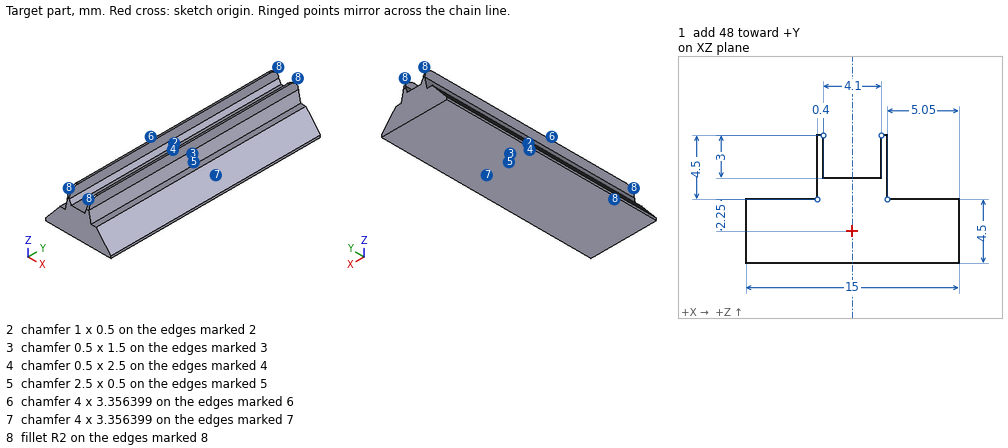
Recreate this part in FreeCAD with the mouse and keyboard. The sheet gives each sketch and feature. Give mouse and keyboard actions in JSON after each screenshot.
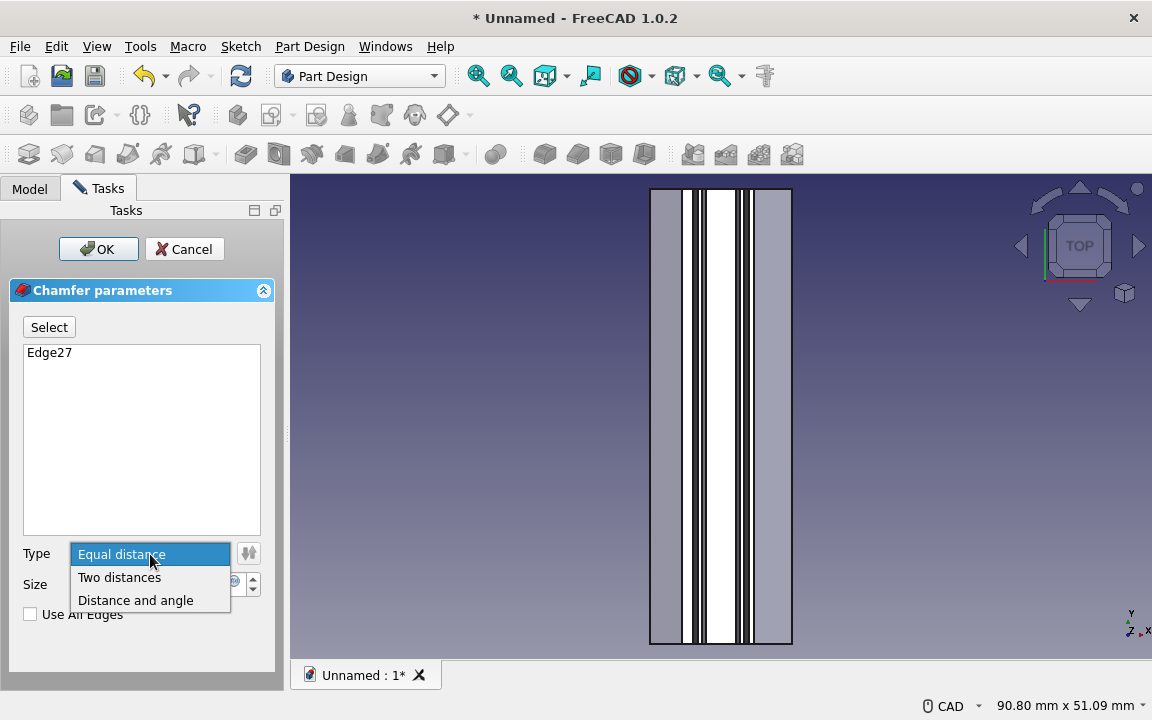
{"action": "left_click", "coordinate": [148, 578]}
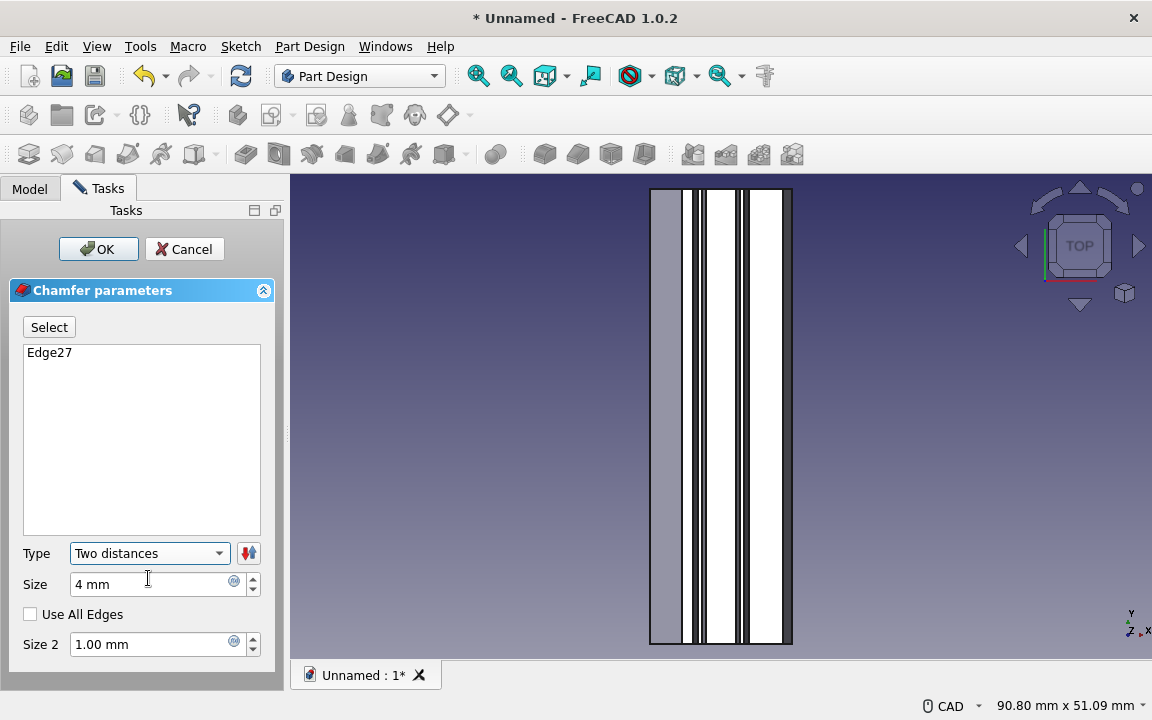
{"action": "triple_click", "coordinate": [158, 644]}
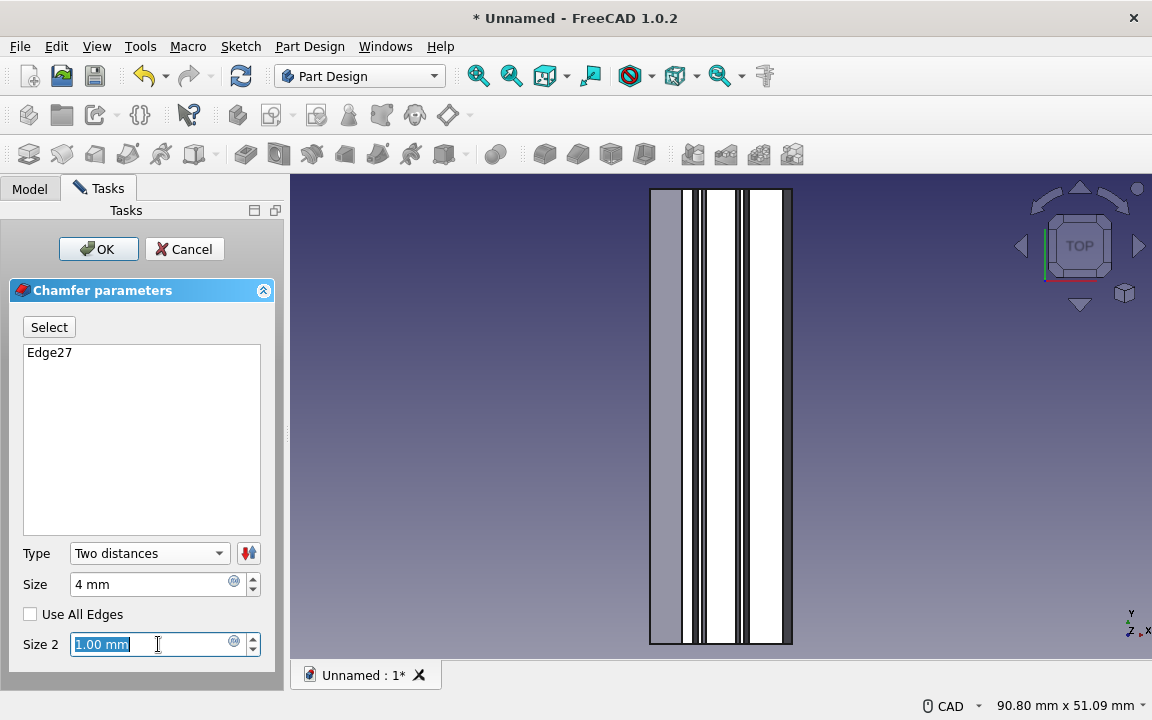
{"action": "type", "text": "3.356399"}
{"action": "key", "text": "Tab"}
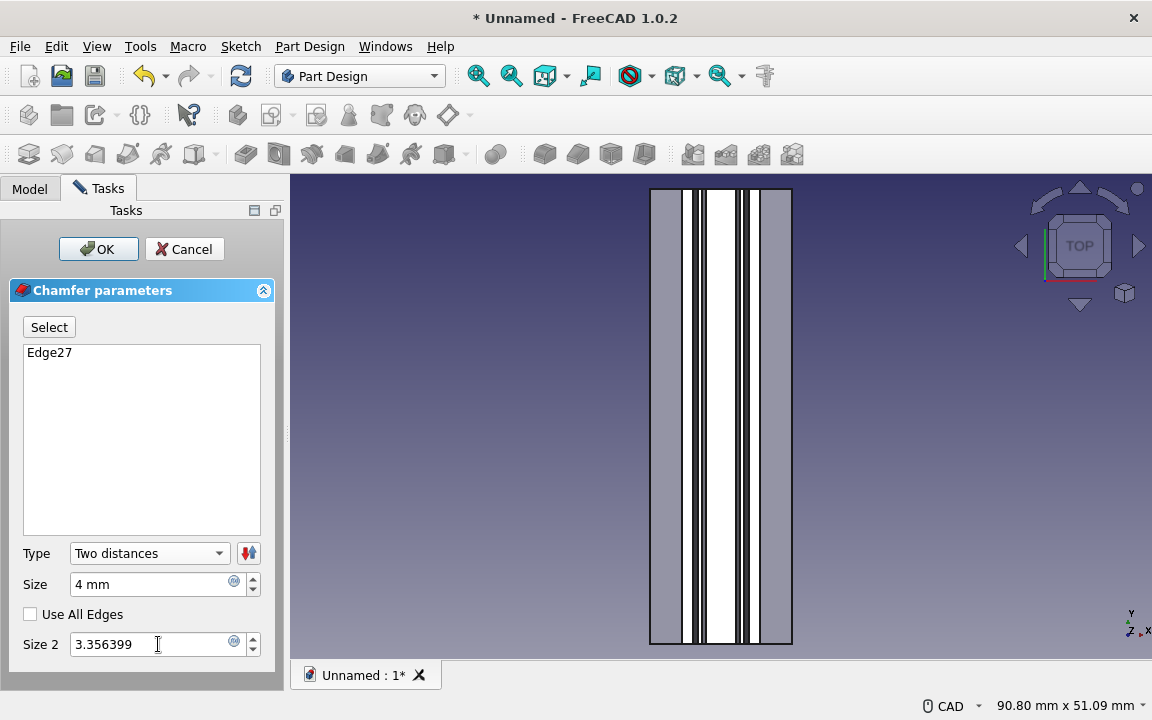
{"action": "left_click", "coordinate": [99, 249]}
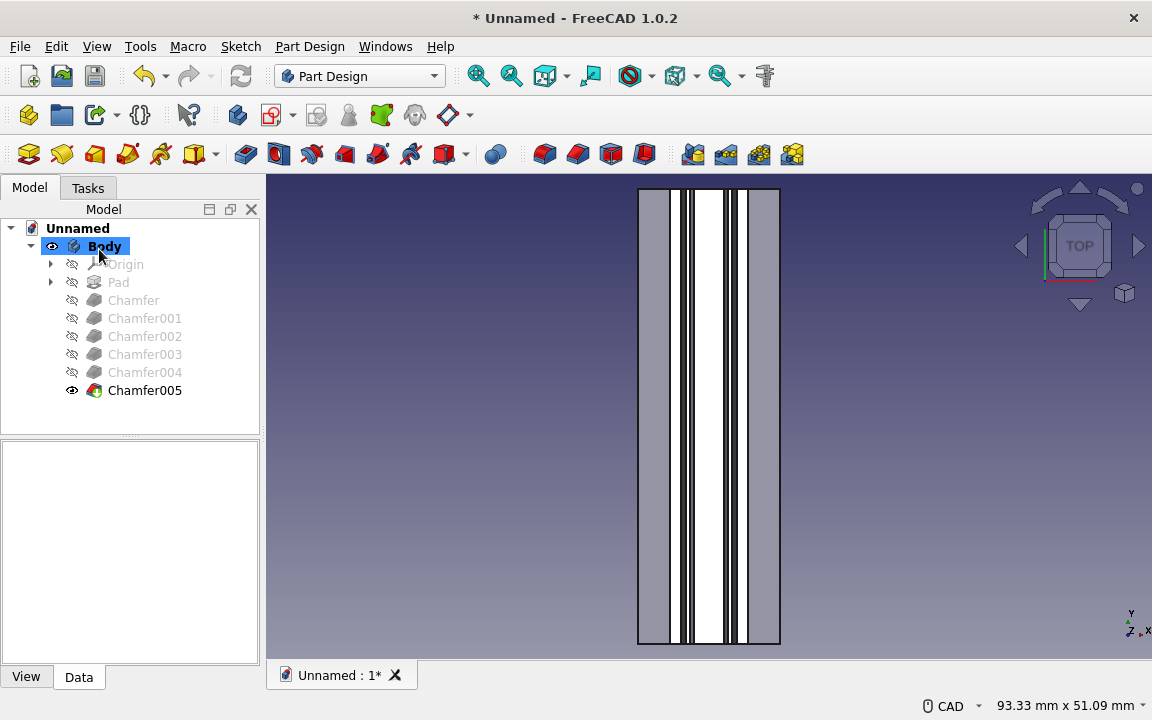
{"action": "key", "text": "0"}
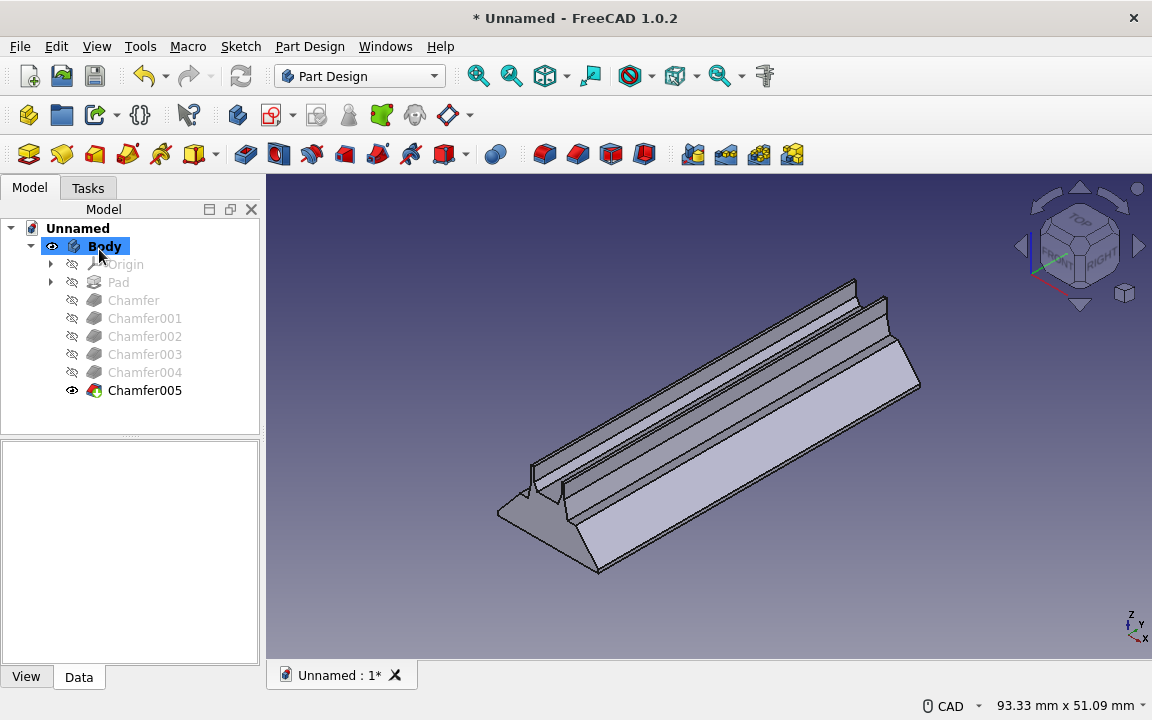
{"action": "scroll", "coordinate": [533, 465], "scroll_direction": "up", "scroll_amount": 12}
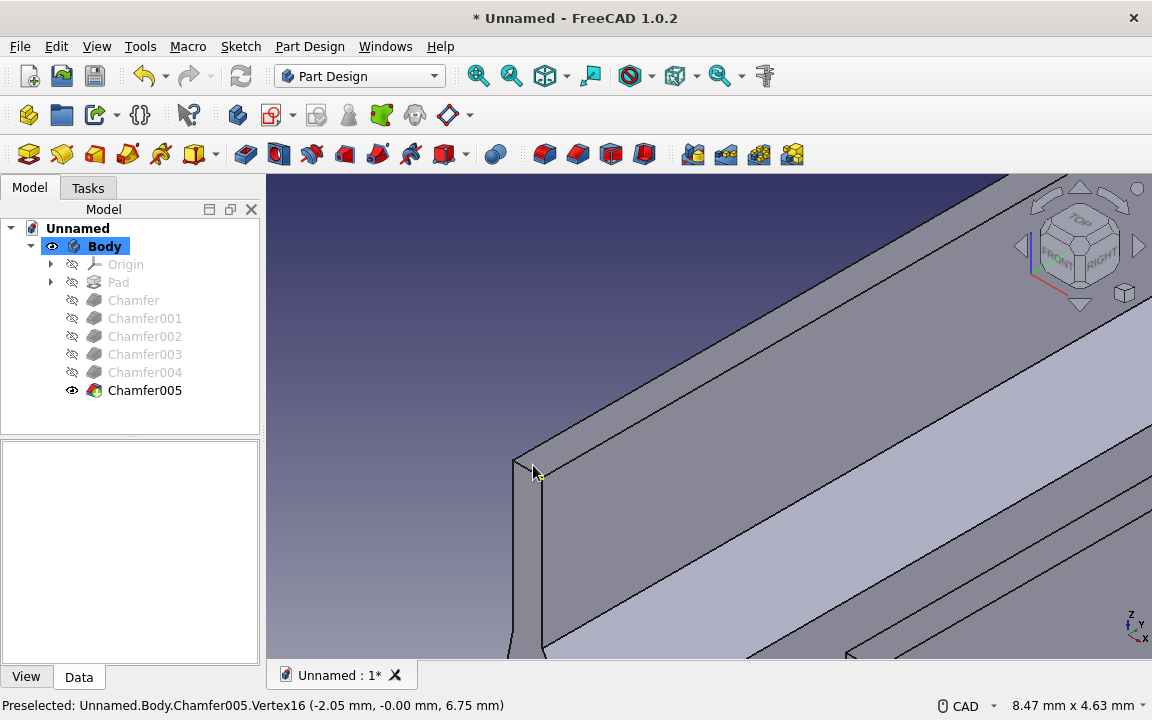
{"action": "left_click", "coordinate": [528, 468]}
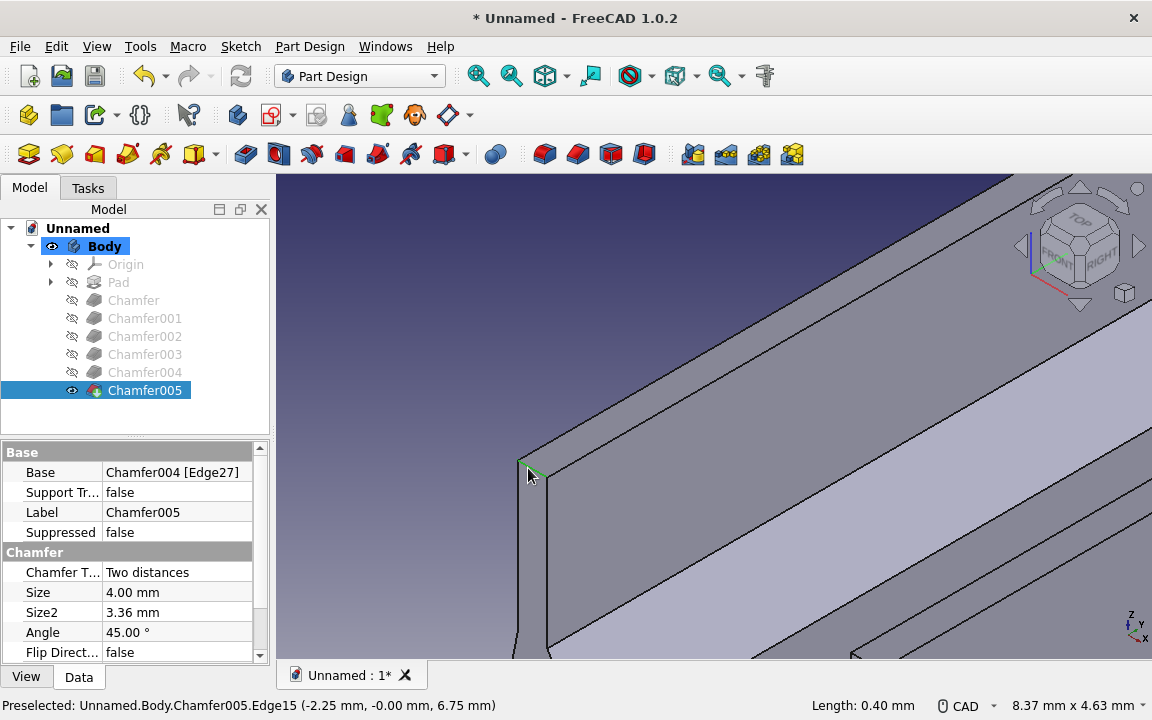
{"action": "key", "text": "v f"}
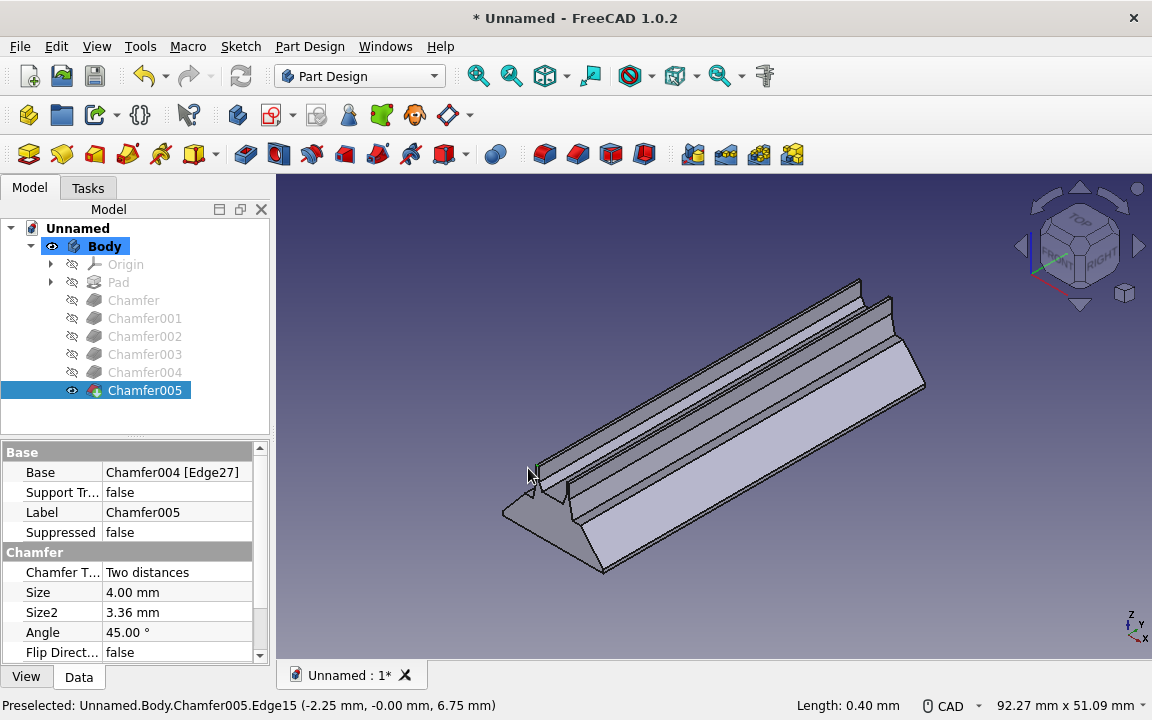
{"action": "key", "text": "2"}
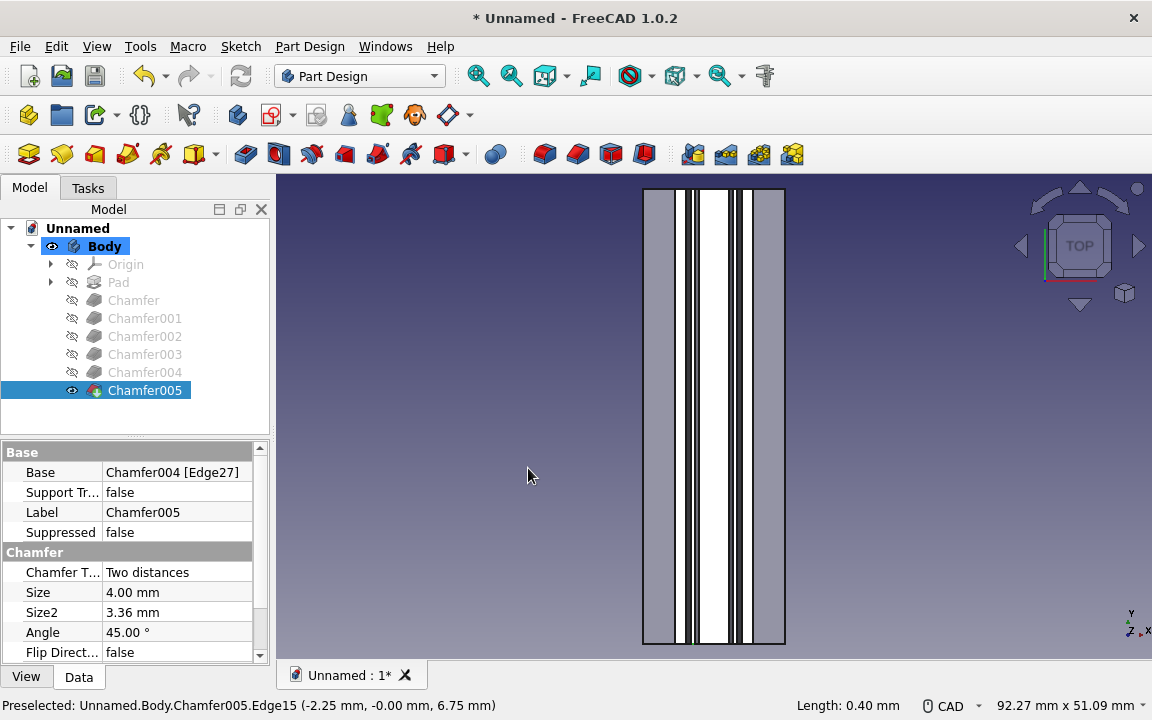
{"action": "key", "text": "1"}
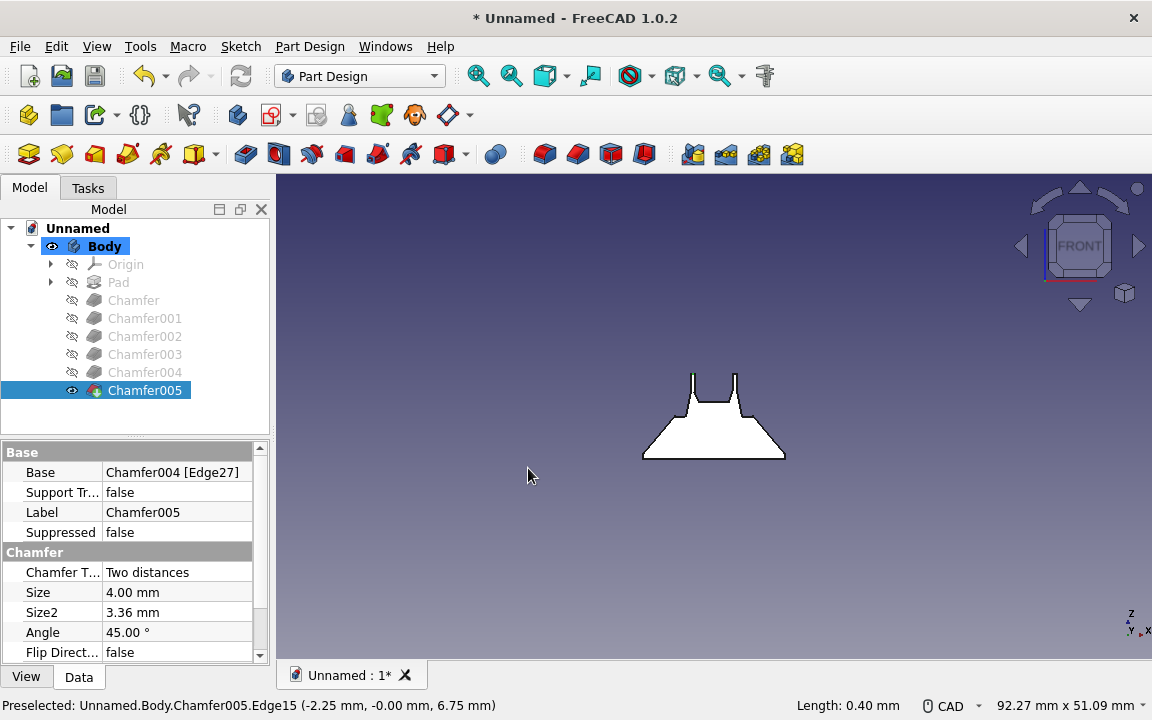
{"action": "left_click", "coordinate": [479, 76]}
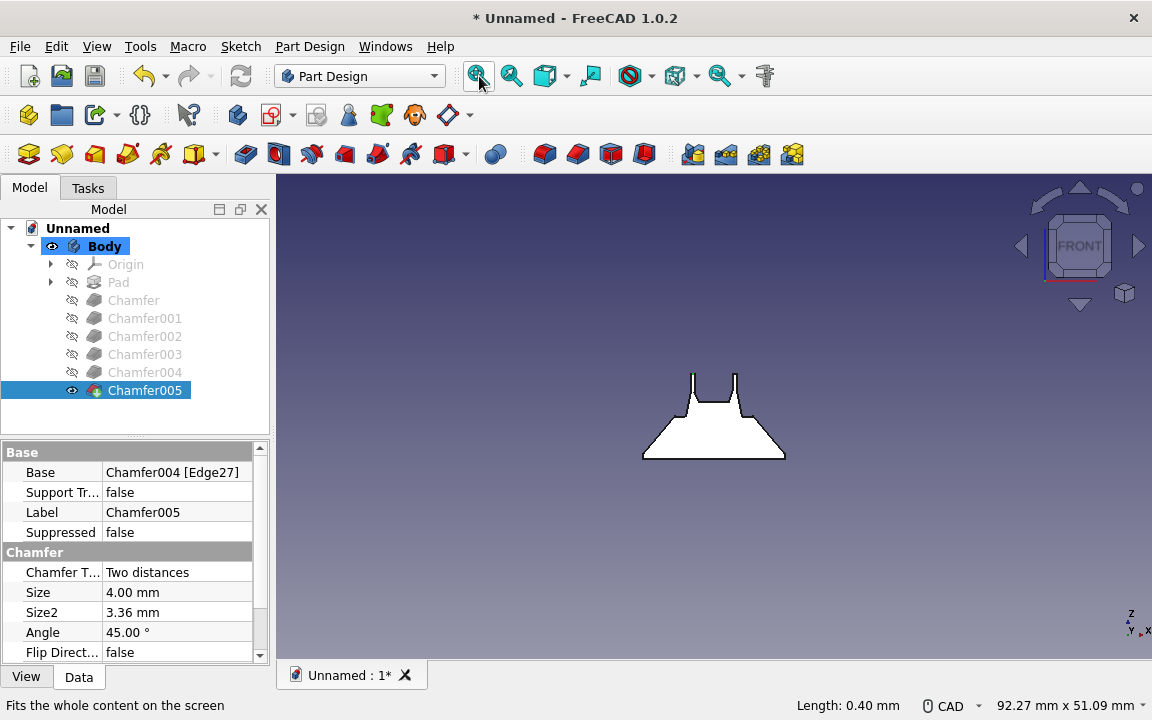
{"action": "scroll", "coordinate": [735, 373], "scroll_direction": "up", "scroll_amount": 12}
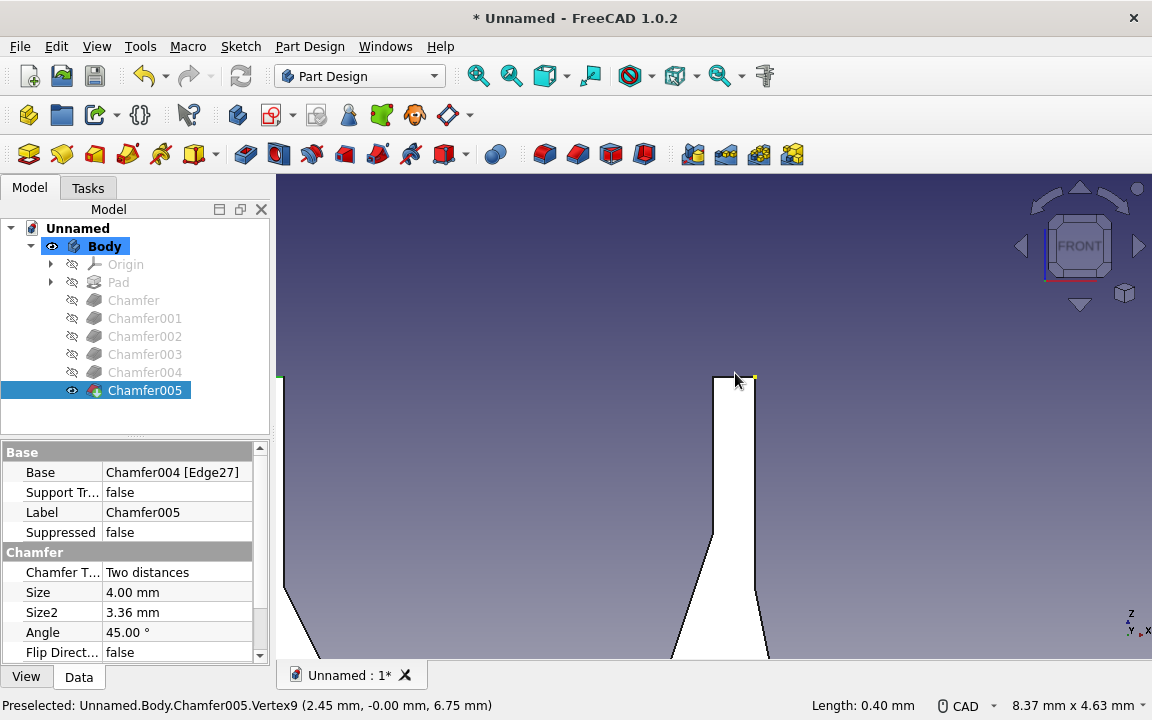
{"action": "left_click", "coordinate": [734, 376], "text": "ctrl"}